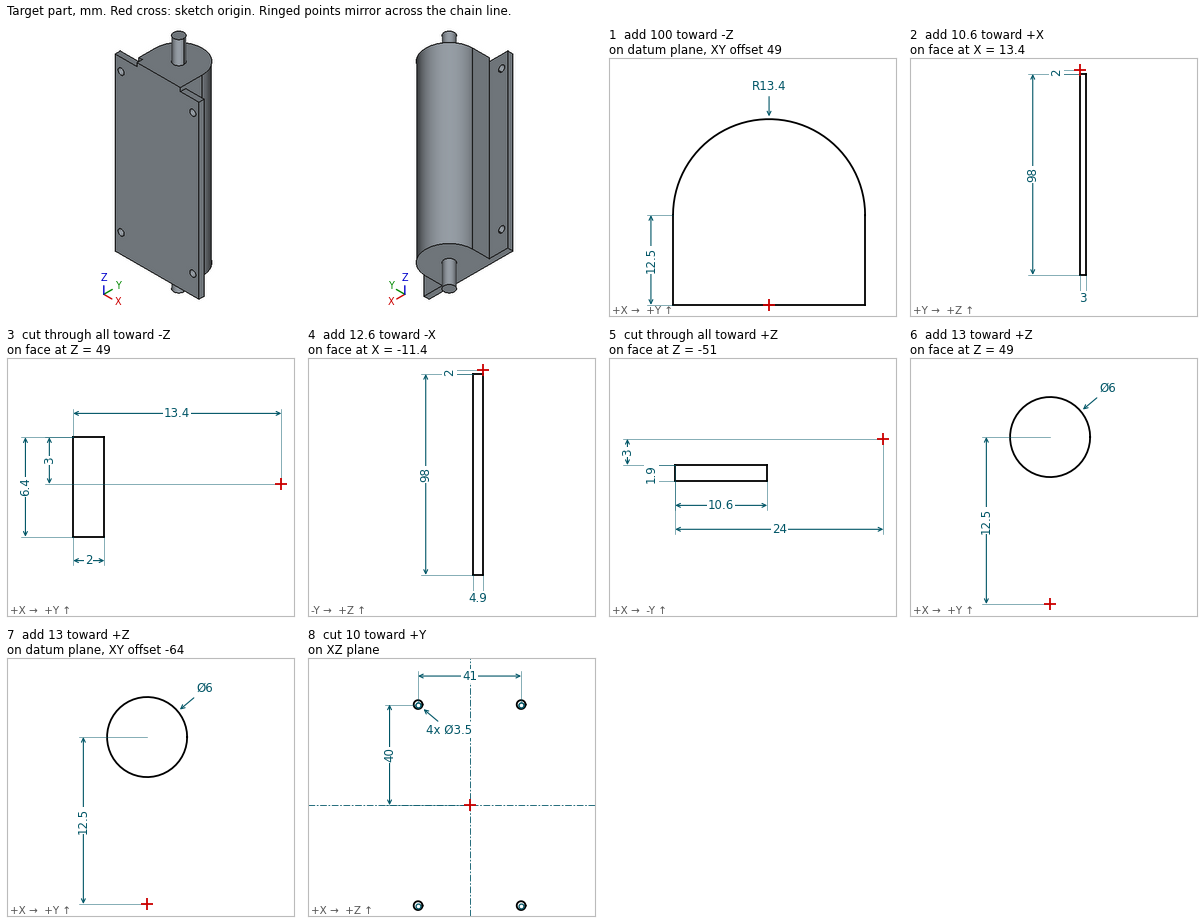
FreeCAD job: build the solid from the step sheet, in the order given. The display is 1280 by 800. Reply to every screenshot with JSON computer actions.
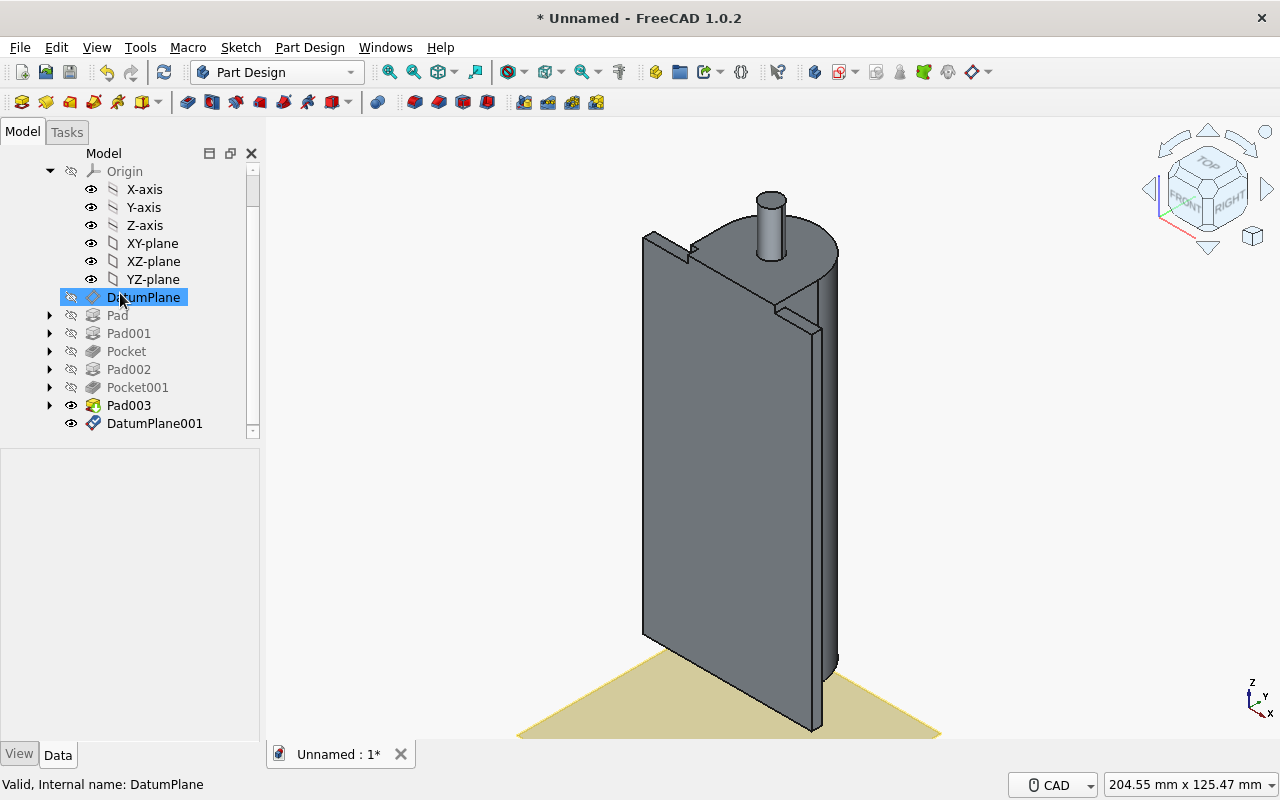
{"action": "left_click", "coordinate": [116, 423]}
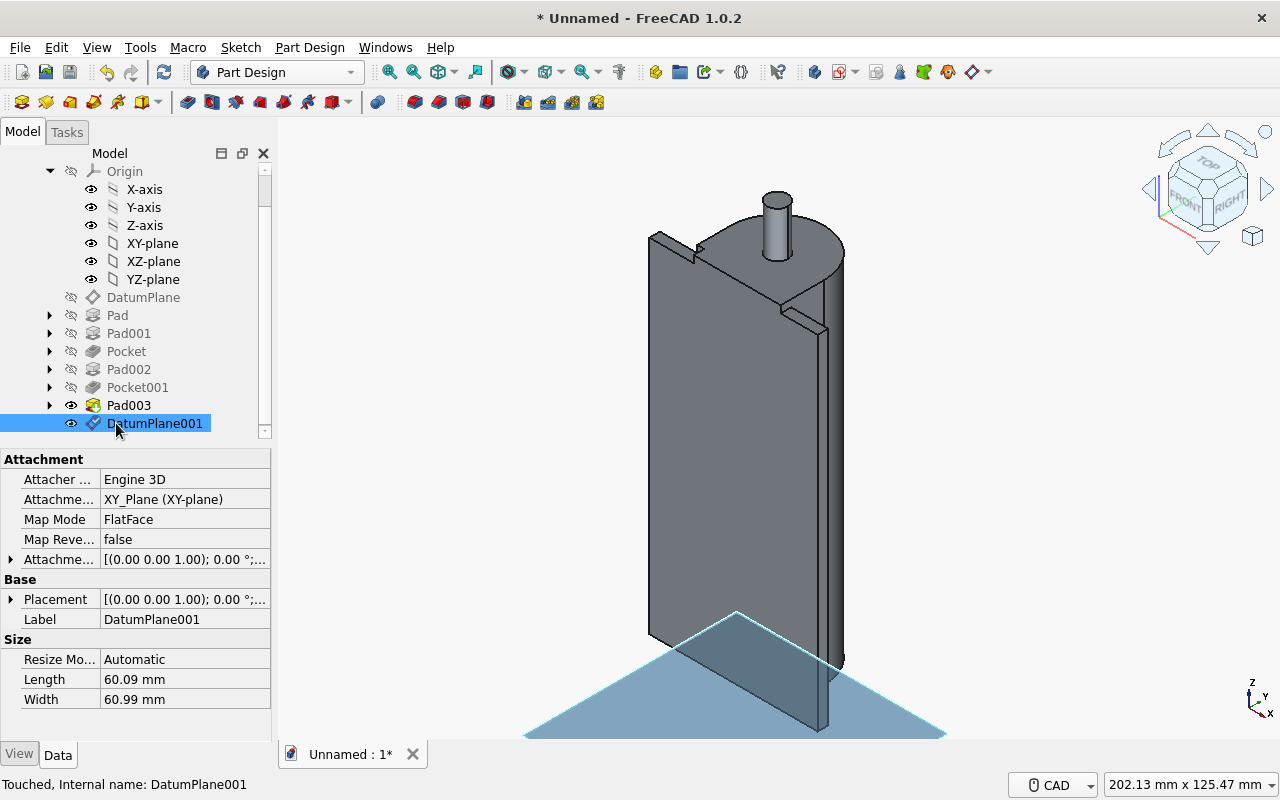
{"action": "left_click", "coordinate": [840, 72]}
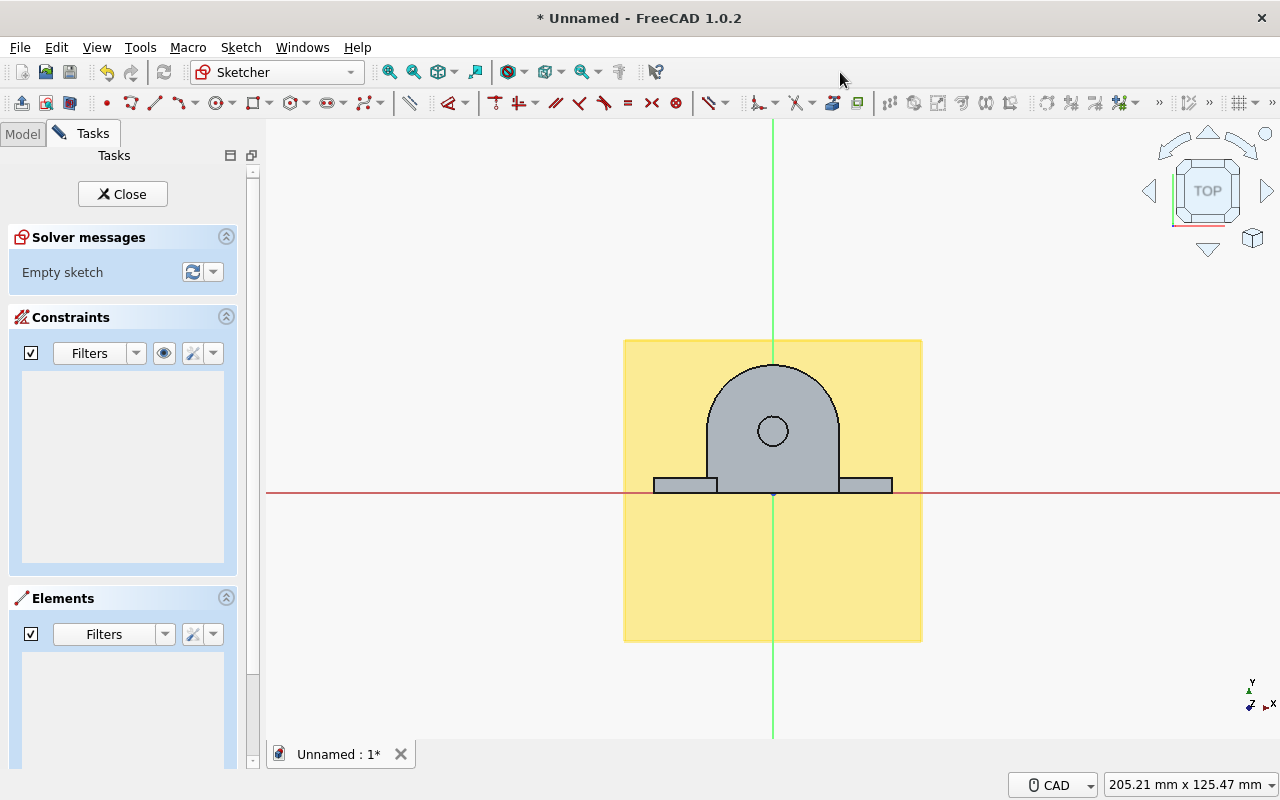
{"action": "left_click", "coordinate": [70, 104]}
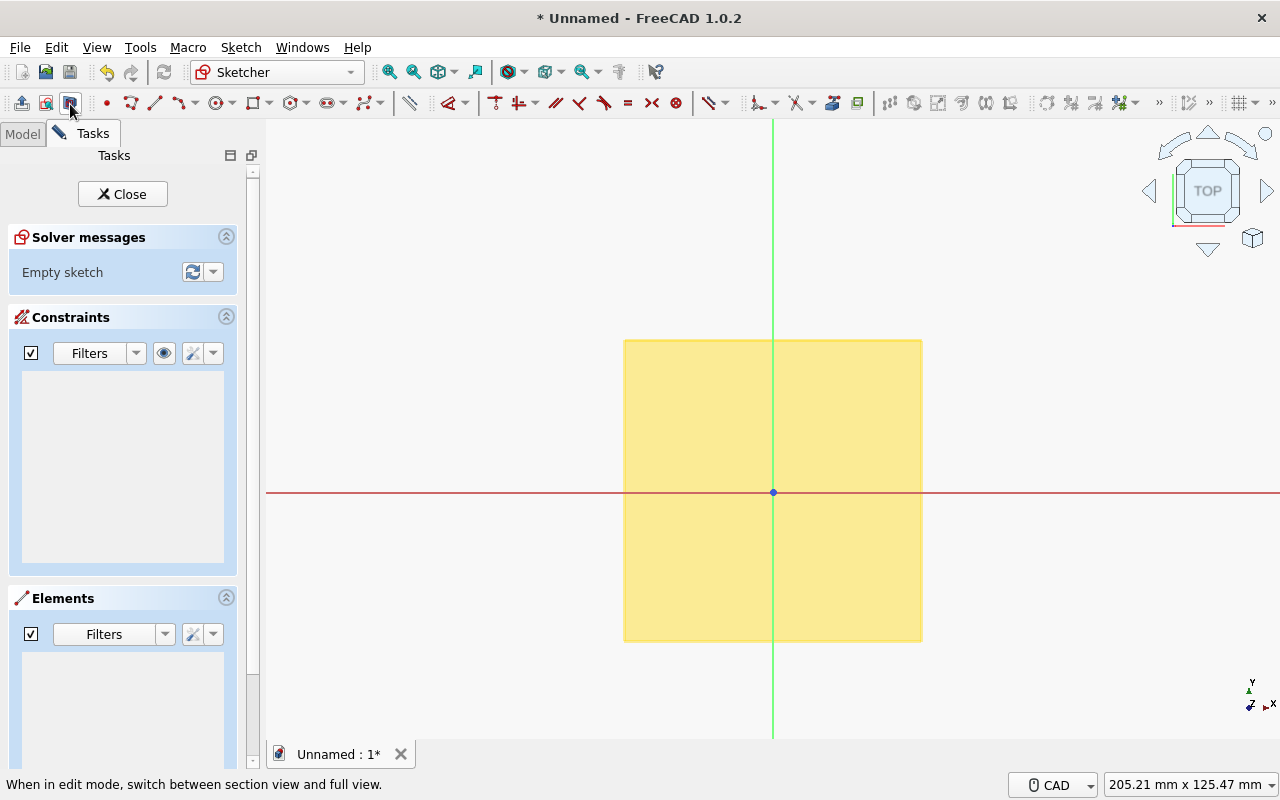
{"action": "scroll", "coordinate": [778, 431], "scroll_direction": "up", "scroll_amount": 13}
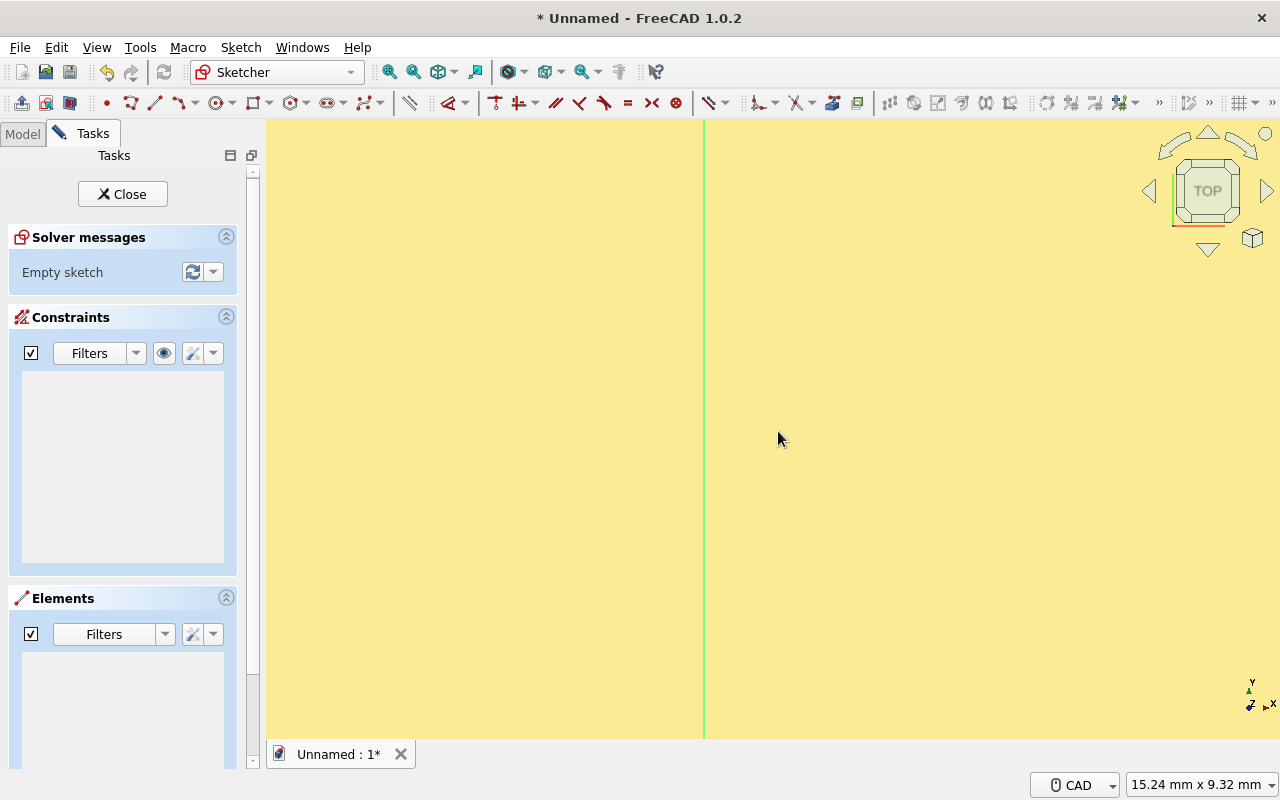
{"action": "left_click", "coordinate": [216, 104]}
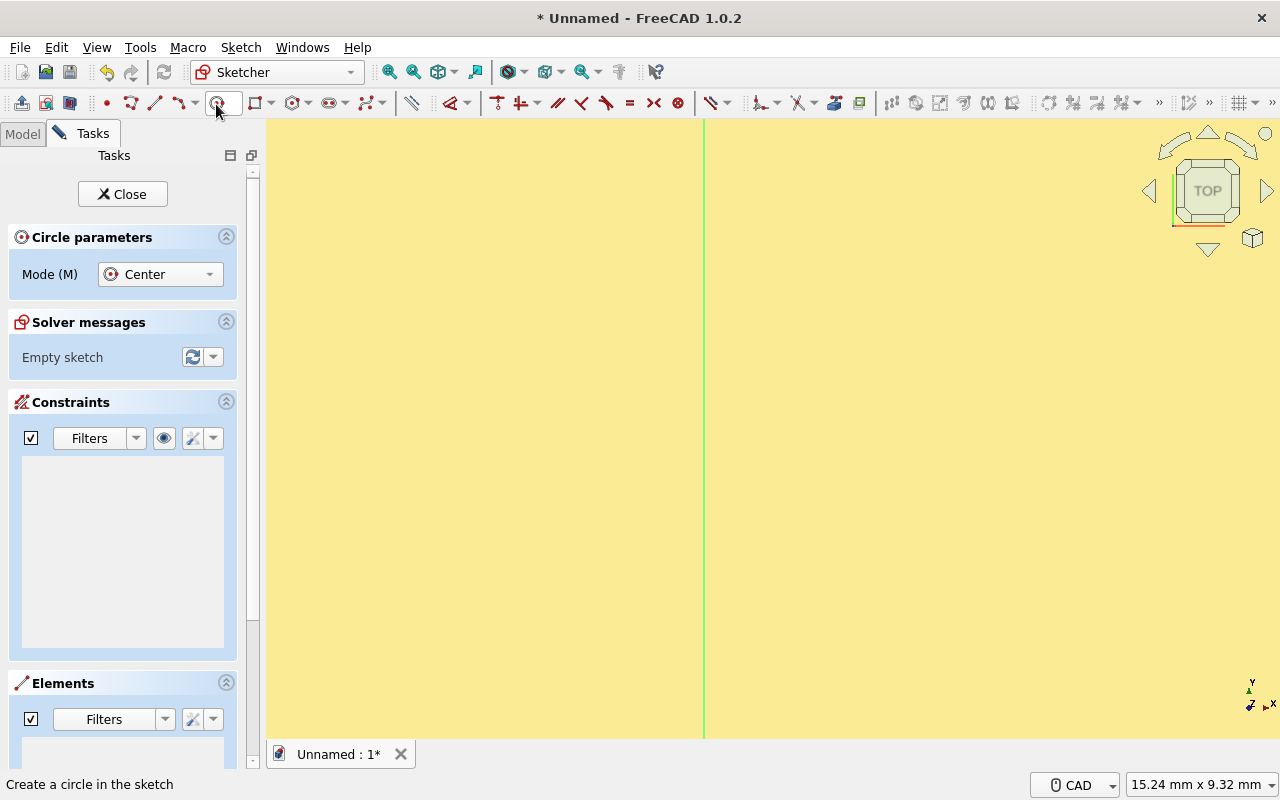
{"action": "left_click", "coordinate": [704, 428]}
{"action": "left_click", "coordinate": [846, 287]}
{"action": "key", "text": "Escape"}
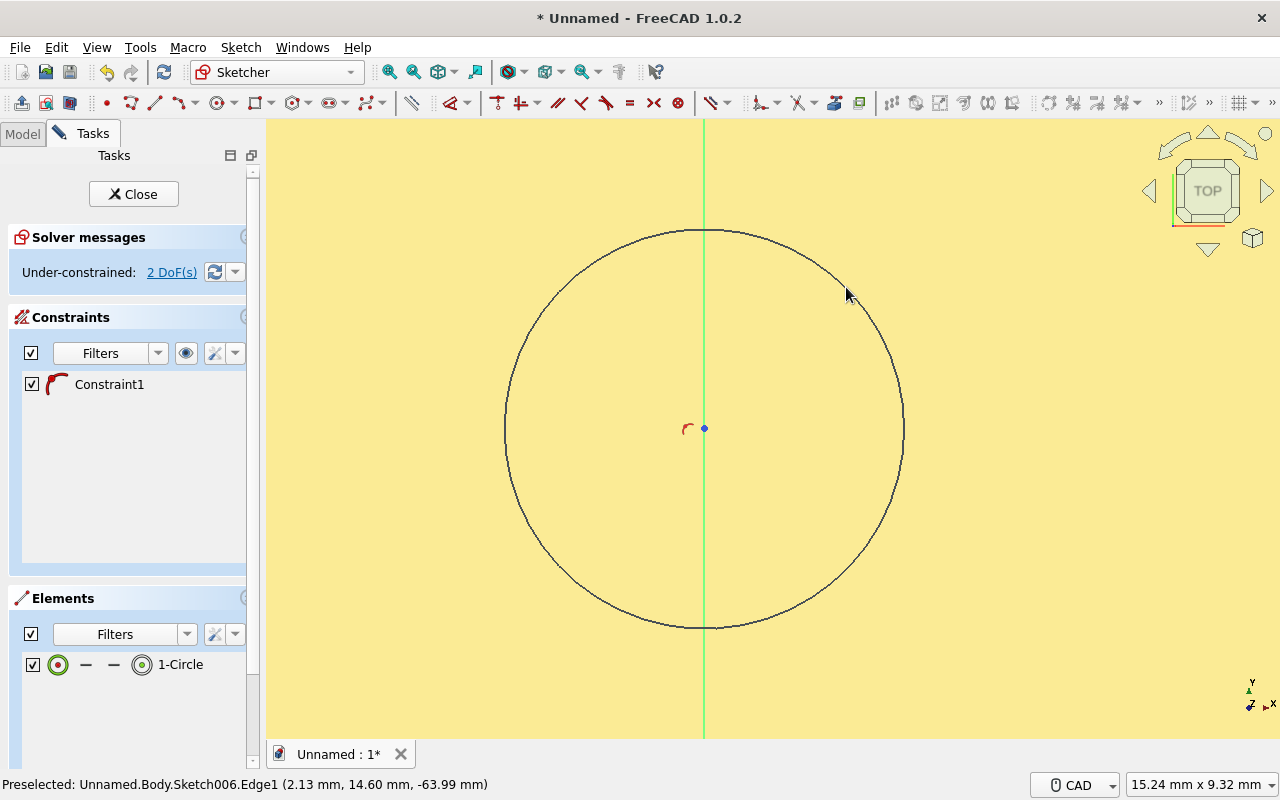
{"action": "left_click", "coordinate": [450, 104]}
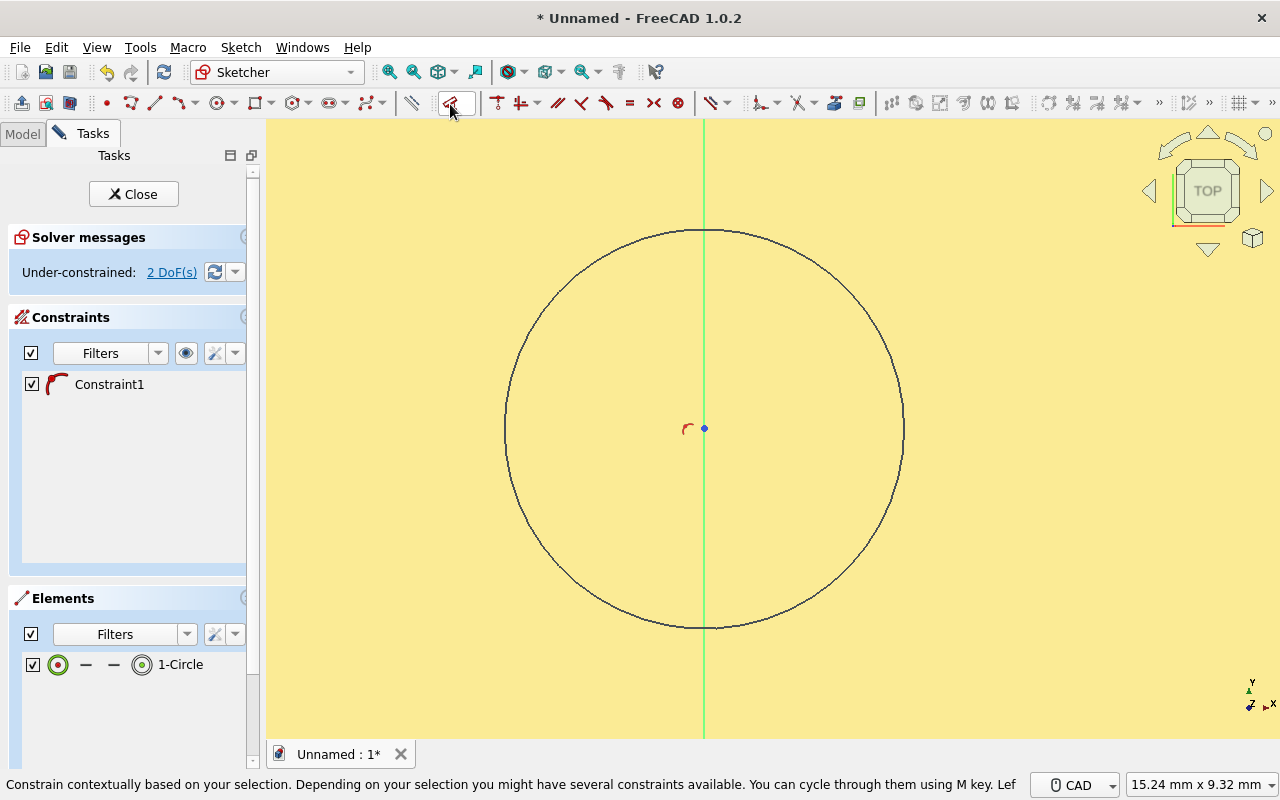
{"action": "left_click", "coordinate": [845, 287]}
{"action": "left_click", "coordinate": [868, 264]}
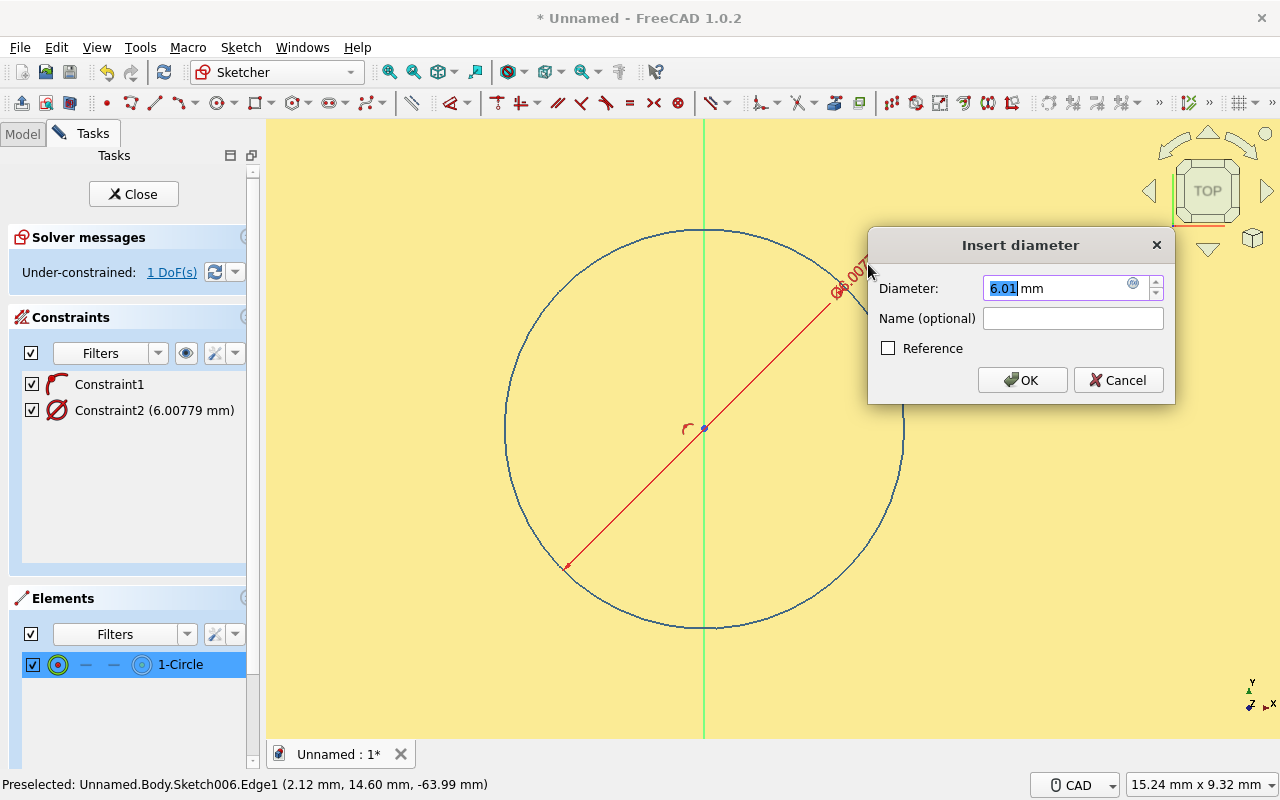
{"action": "type", "text": "6"}
{"action": "key", "text": "Return"}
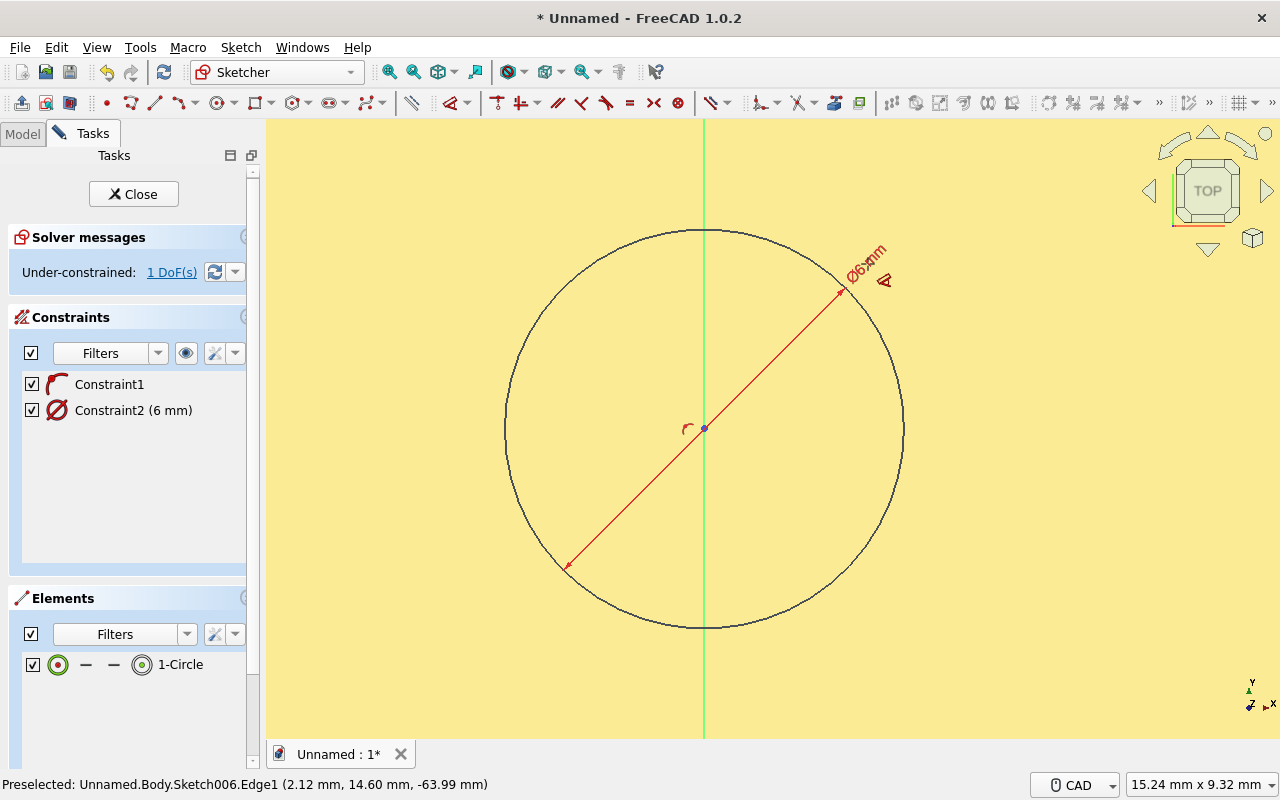
{"action": "left_click", "coordinate": [704, 429]}
{"action": "left_click", "coordinate": [738, 570]}